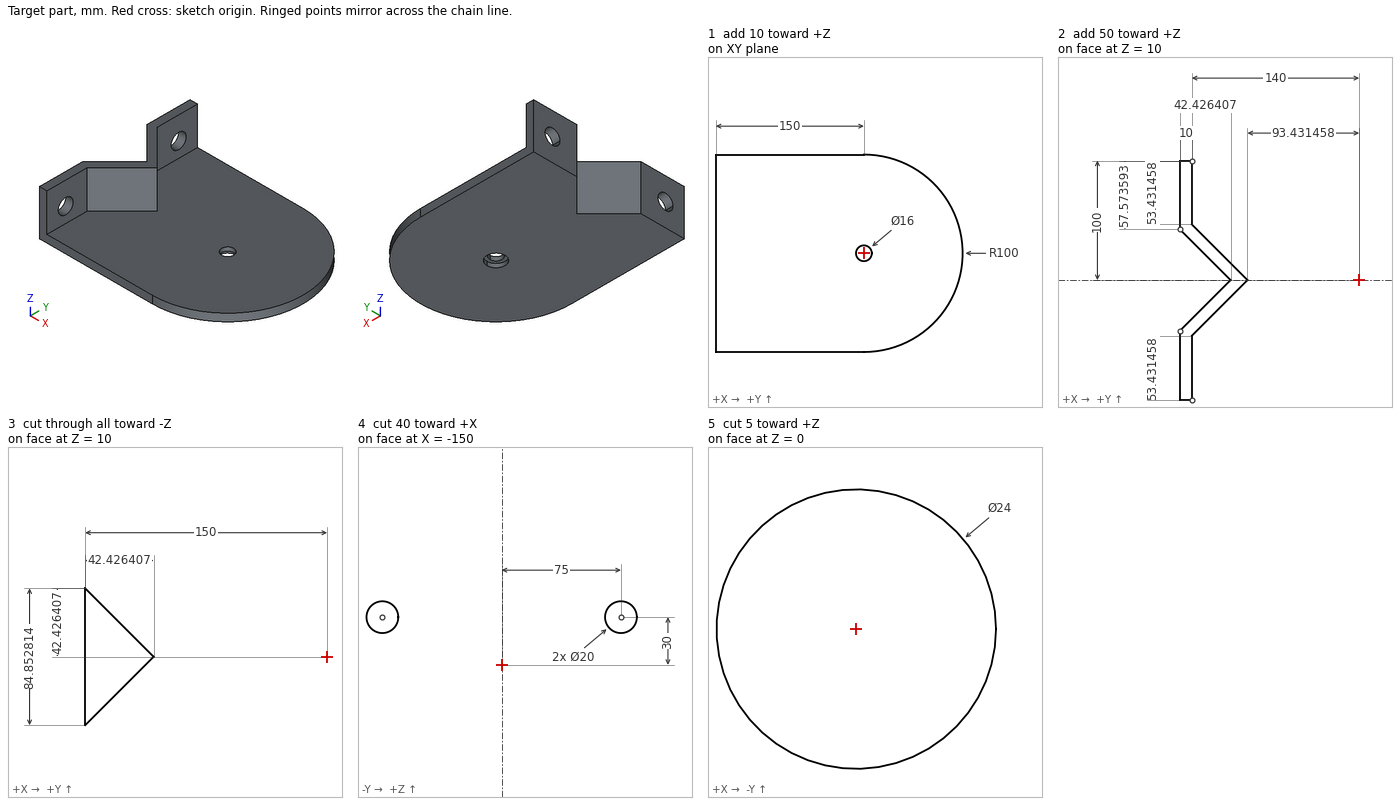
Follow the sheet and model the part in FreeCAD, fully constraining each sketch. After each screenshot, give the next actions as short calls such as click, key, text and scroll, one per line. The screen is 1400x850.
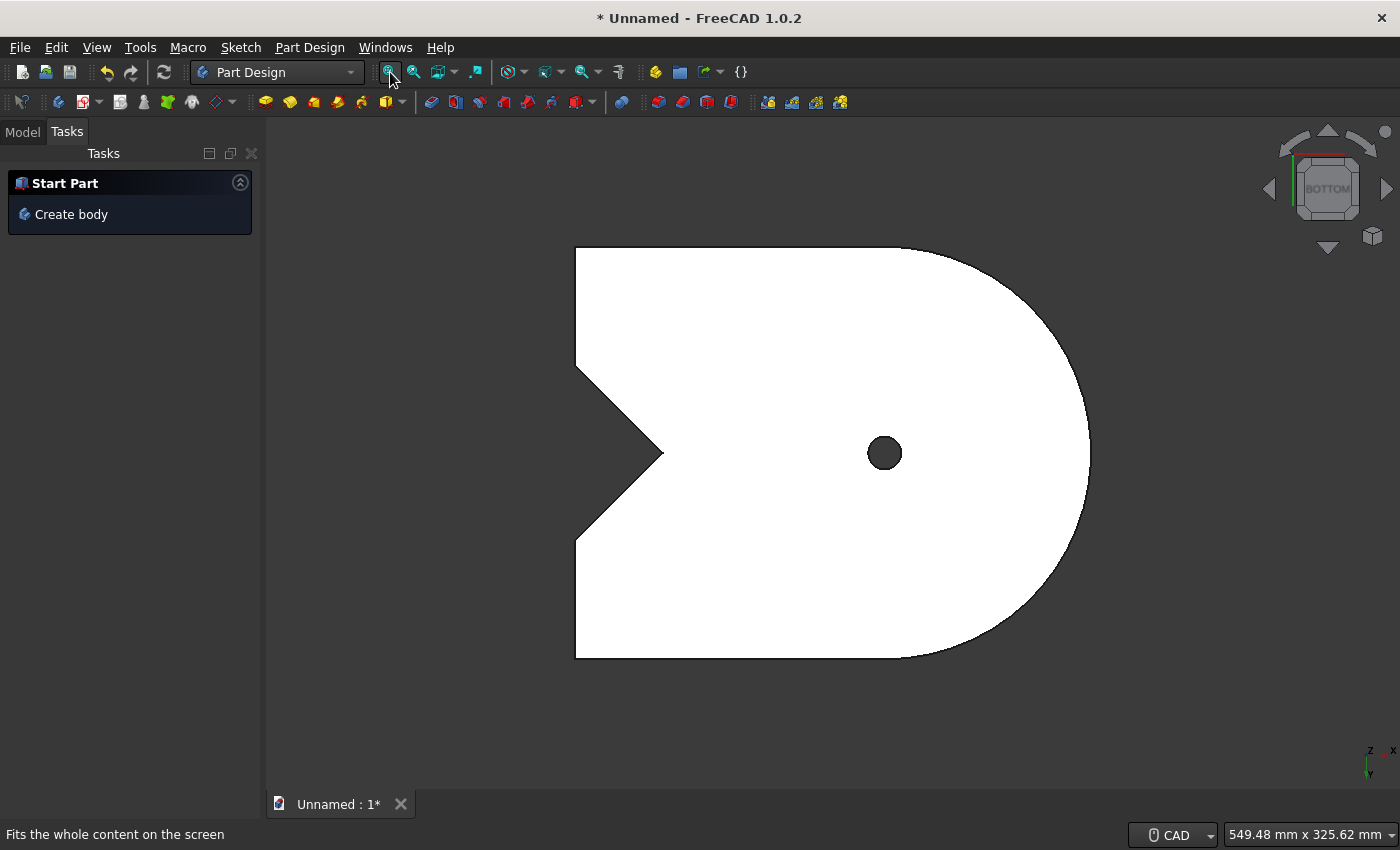
click(759, 511)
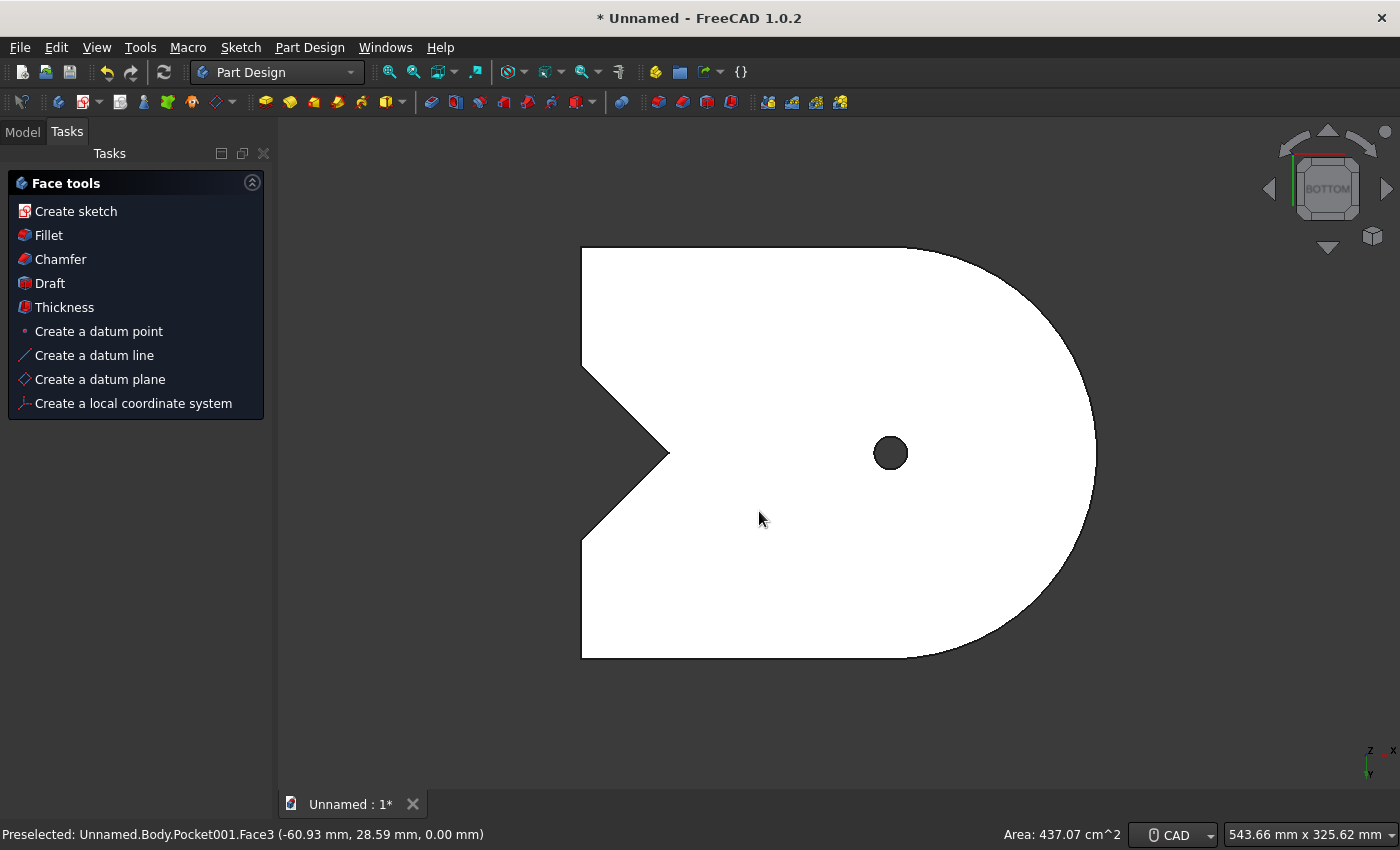
click(84, 102)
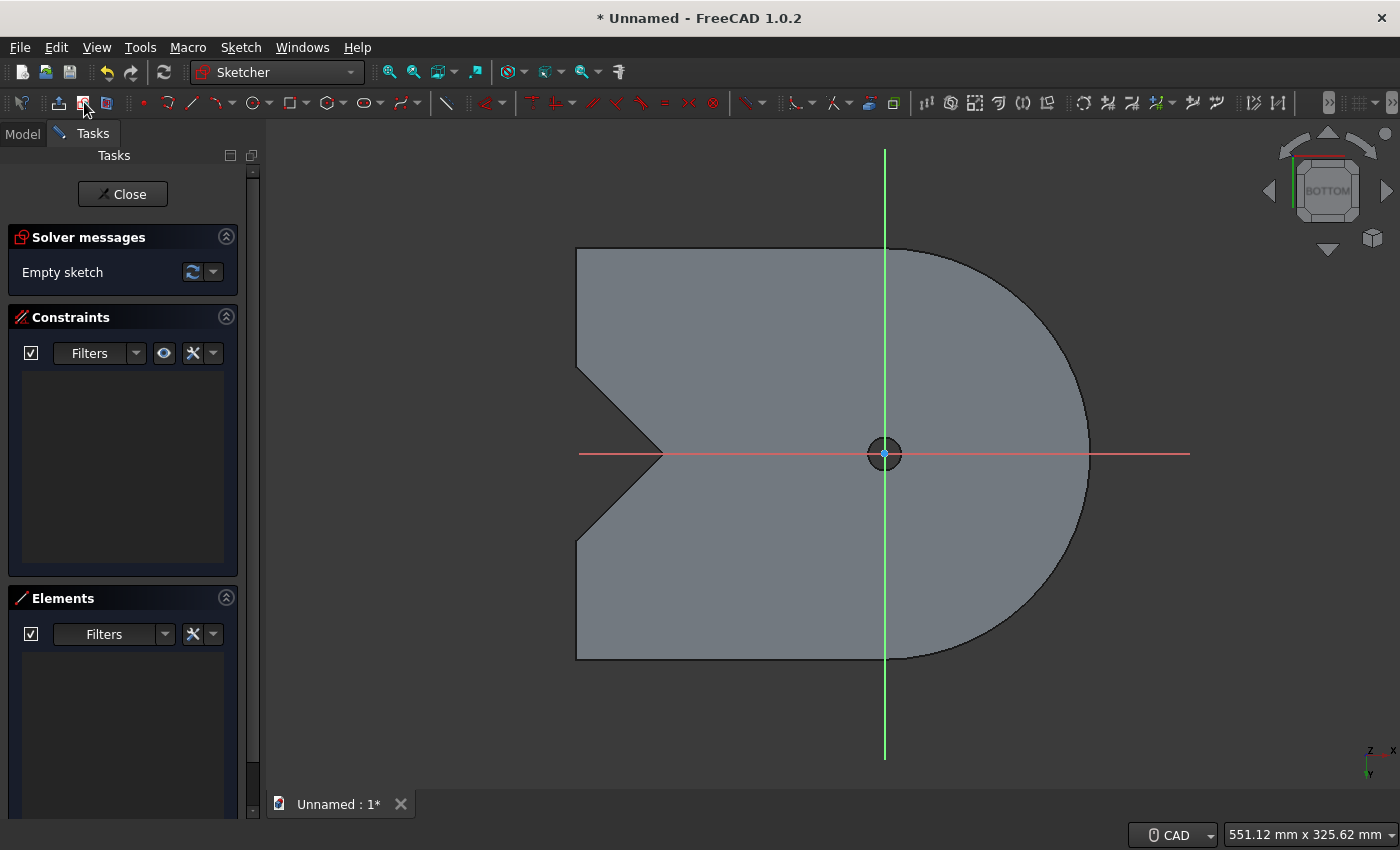
scroll(900, 454, up, 11)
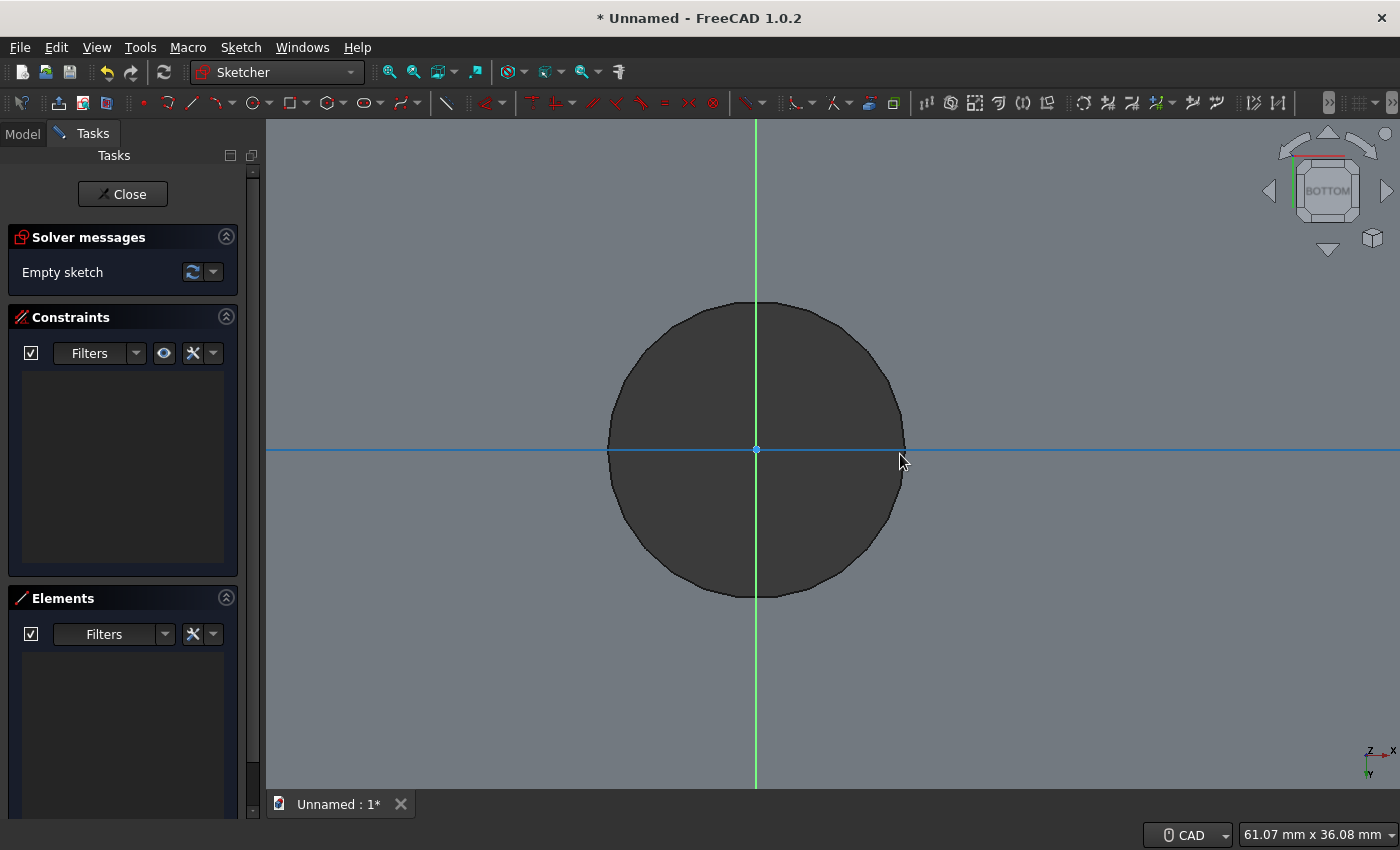
click(254, 104)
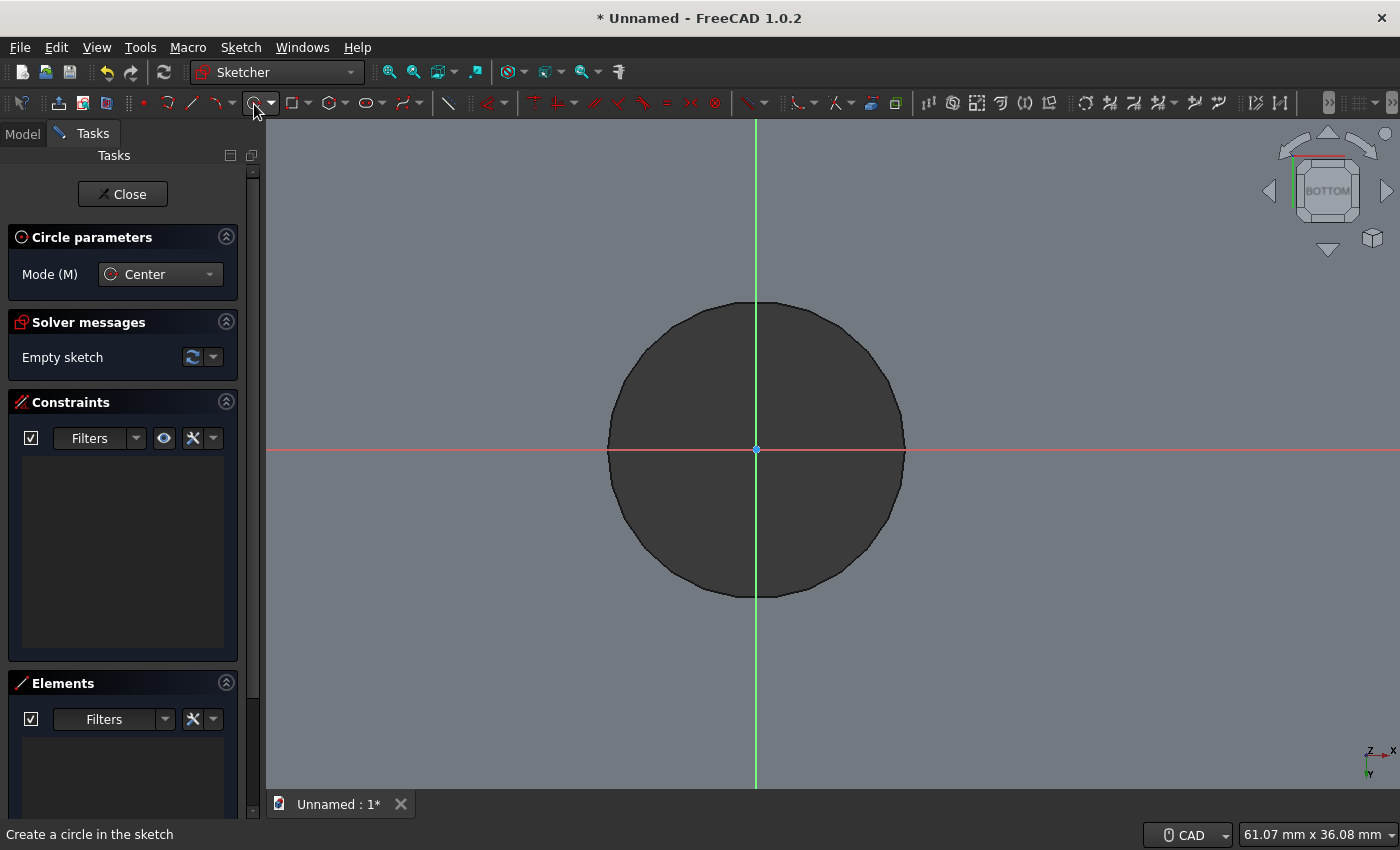
click(756, 450)
click(914, 292)
key(Escape)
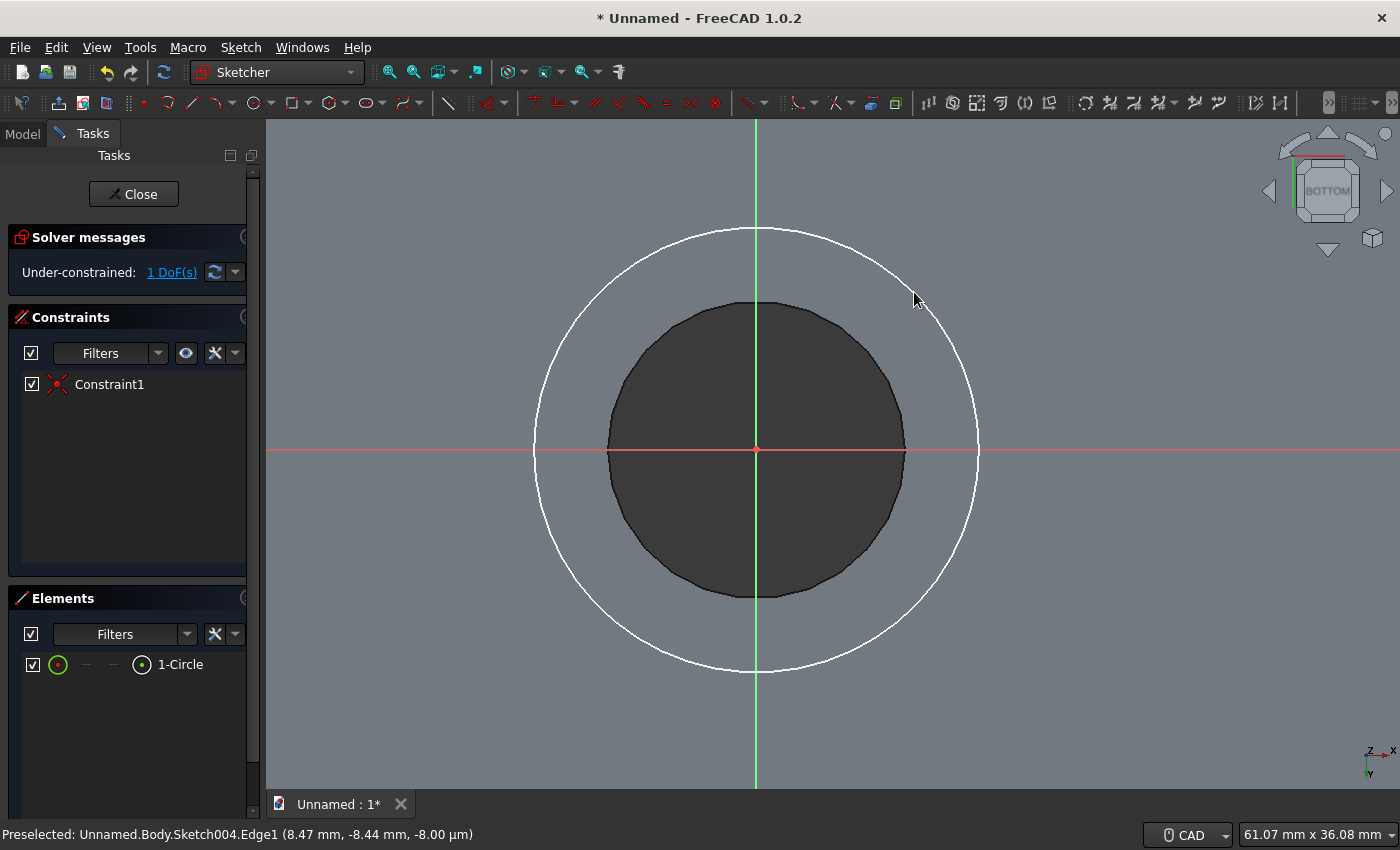
click(488, 104)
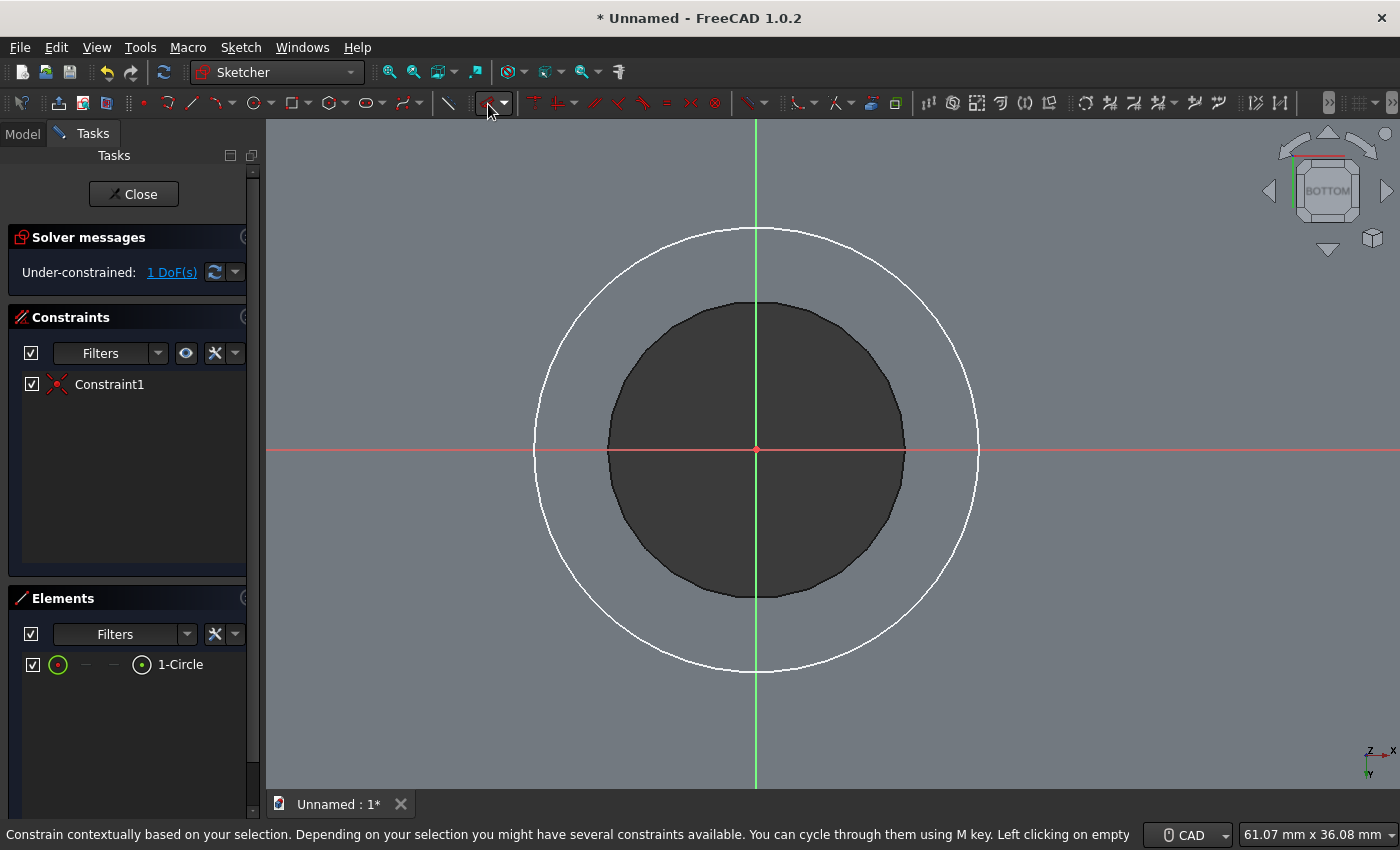
click(913, 292)
click(936, 269)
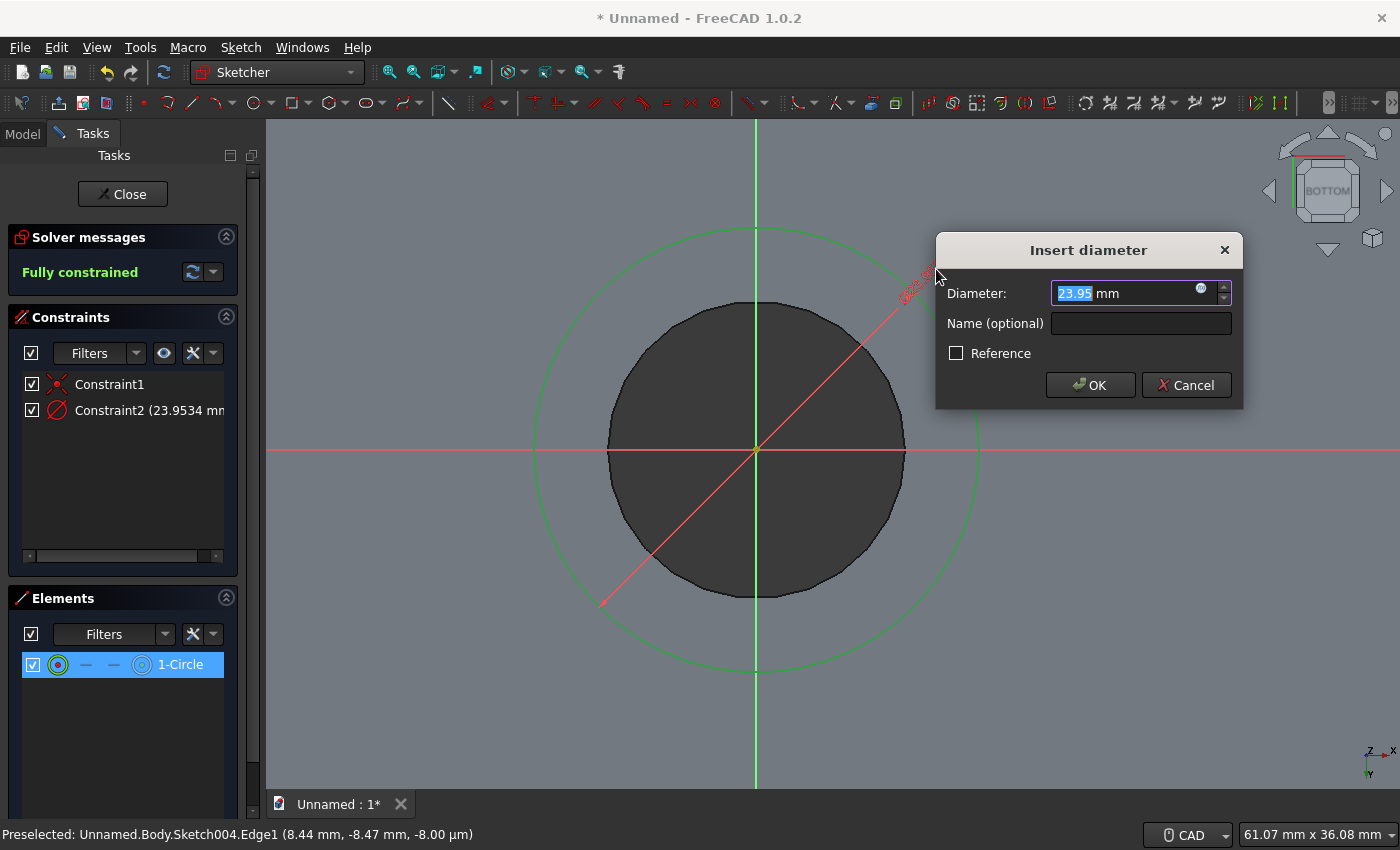
text(24)
key(Return)
key(Escape)